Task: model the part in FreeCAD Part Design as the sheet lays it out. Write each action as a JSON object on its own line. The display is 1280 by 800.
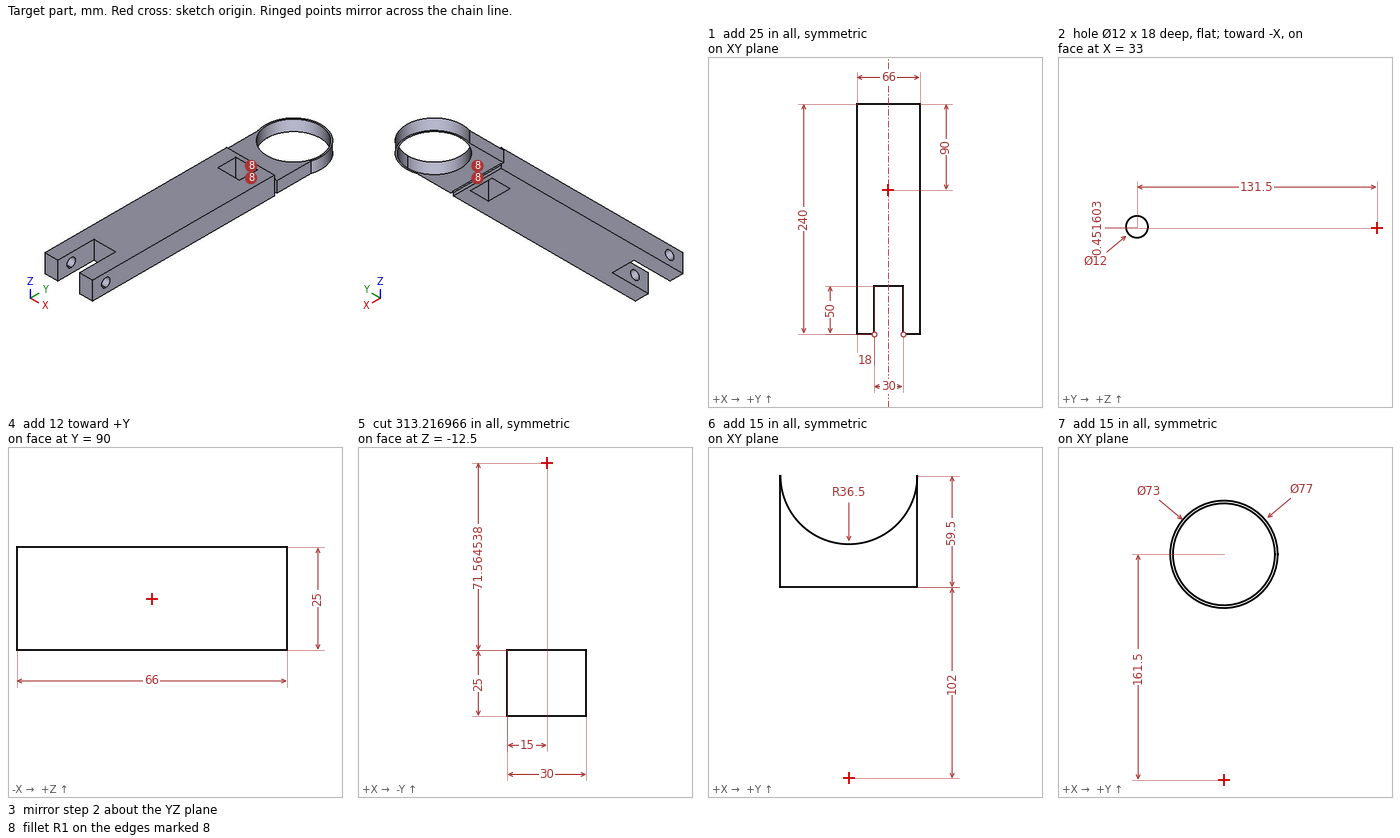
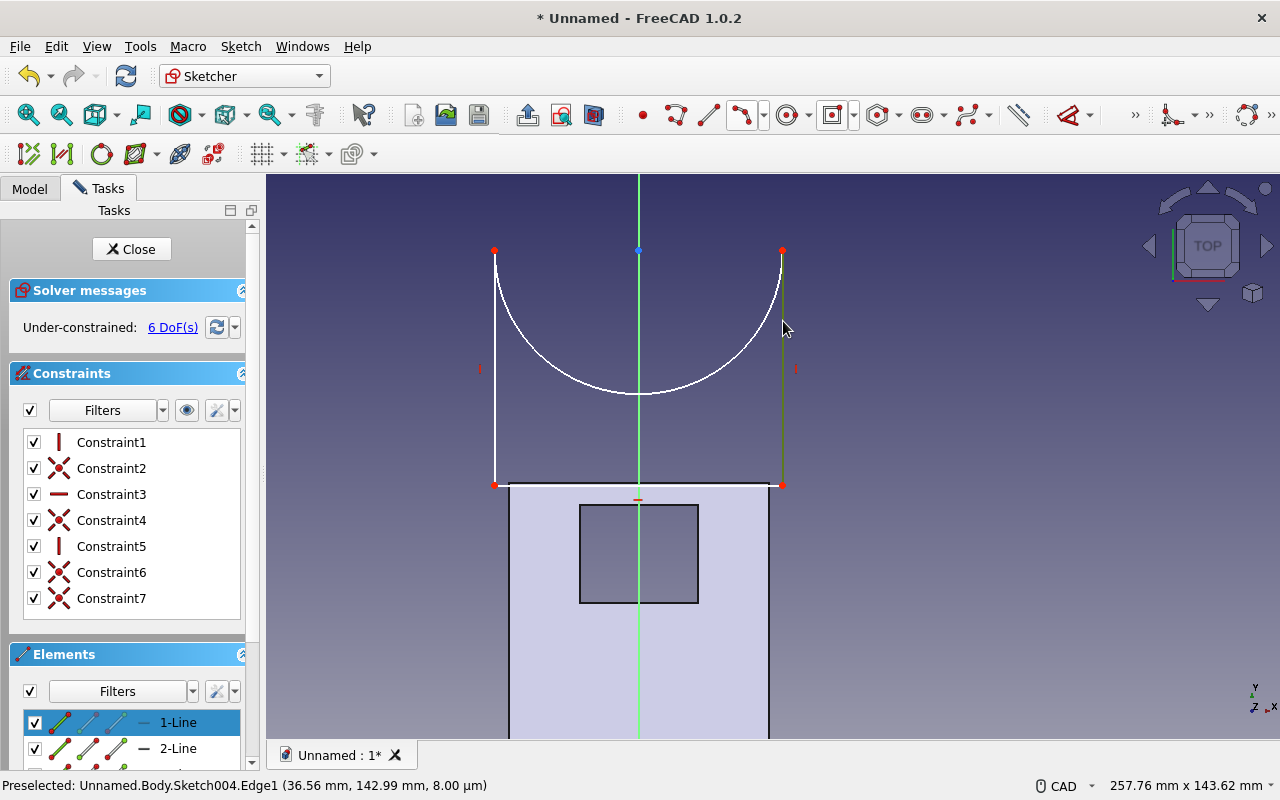
{"action": "left_click", "coordinate": [554, 367]}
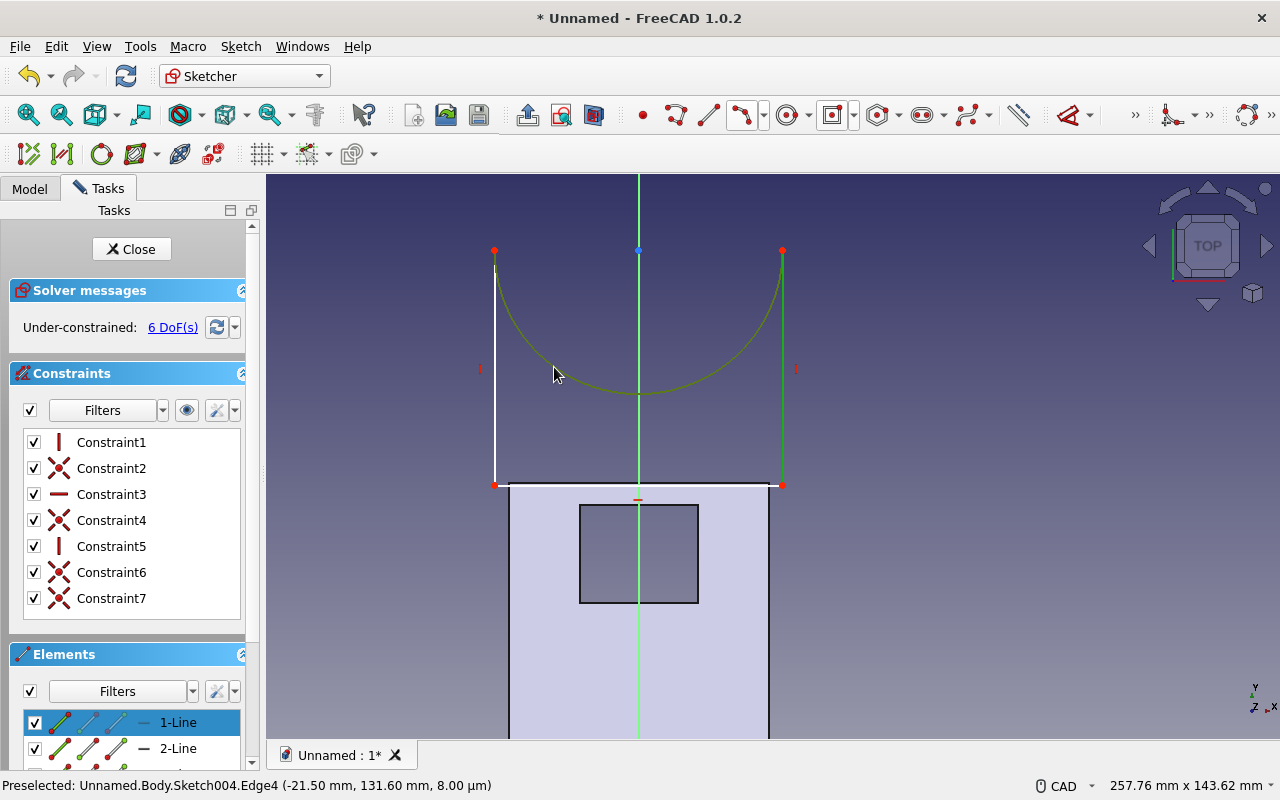
{"action": "key", "text": "t"}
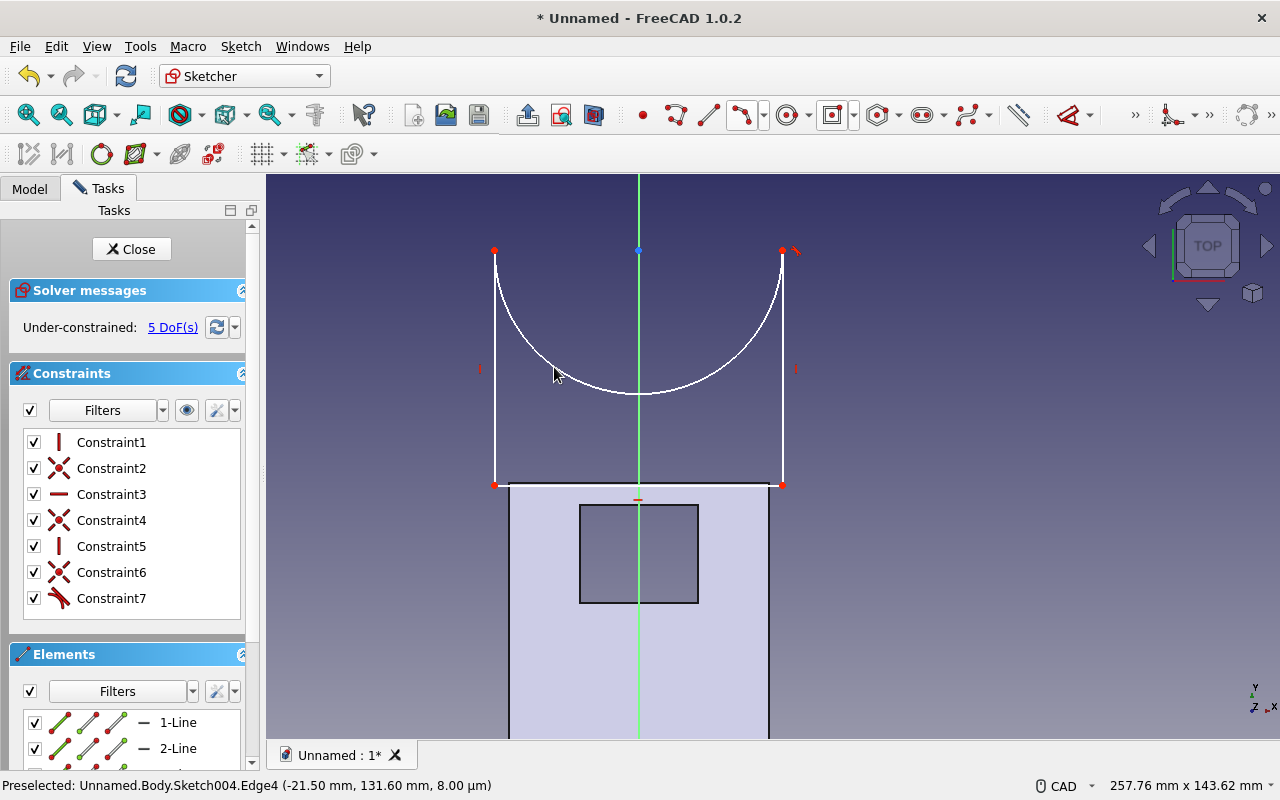
{"action": "left_click", "coordinate": [495, 415]}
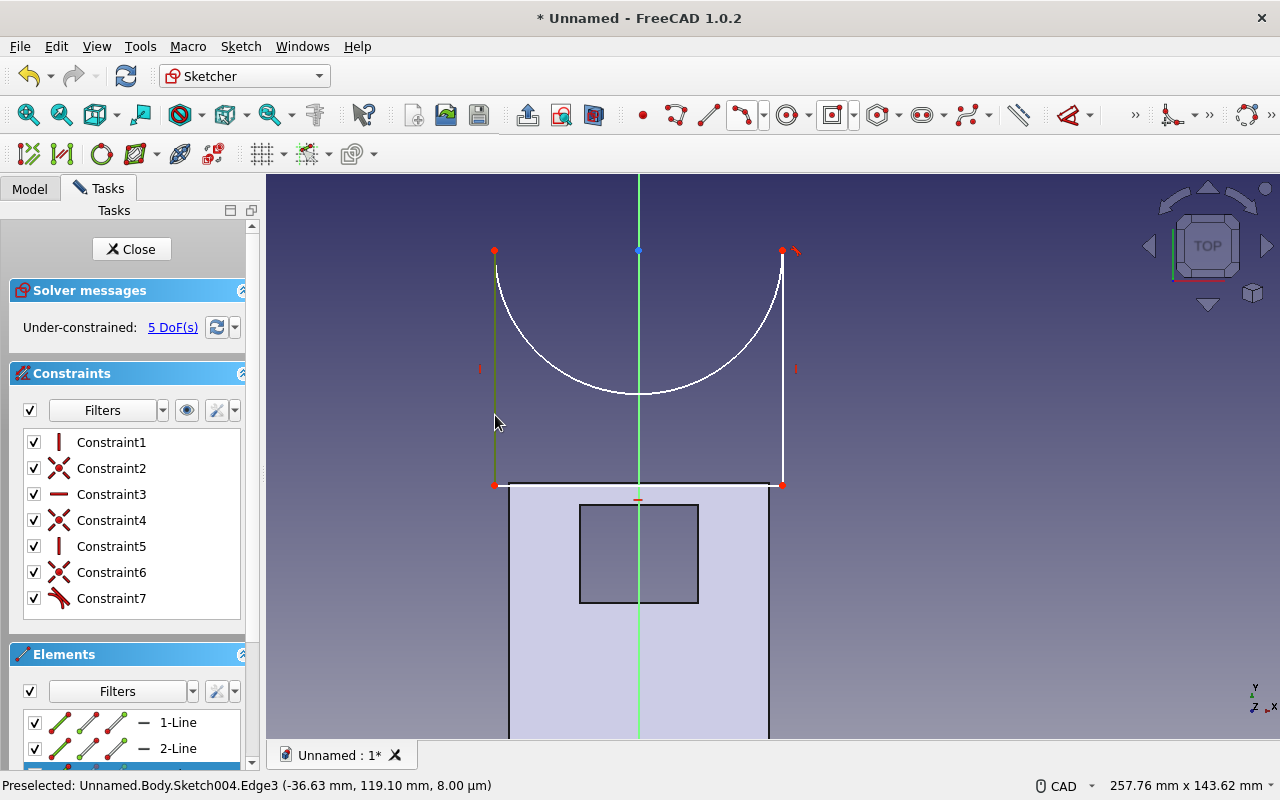
{"action": "left_click", "coordinate": [554, 367]}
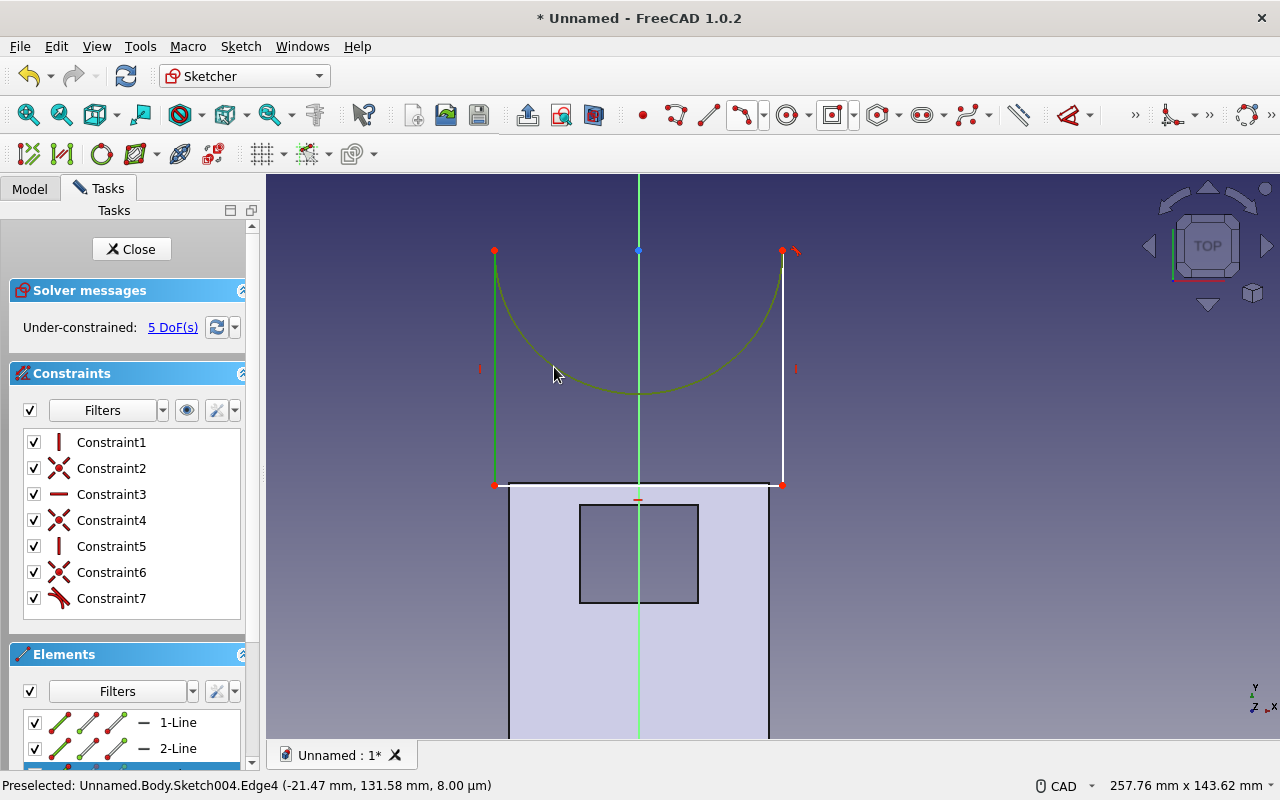
{"action": "key", "text": "t"}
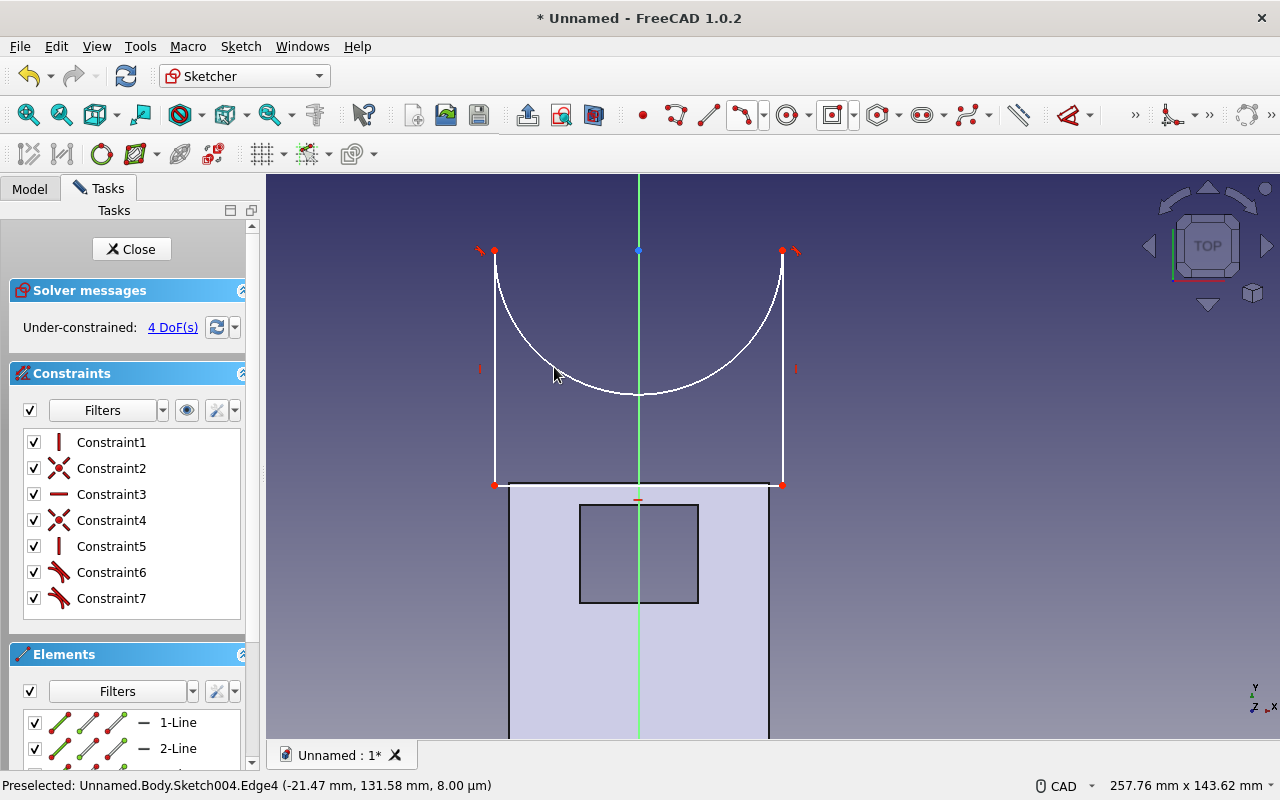
{"action": "left_click", "coordinate": [639, 251]}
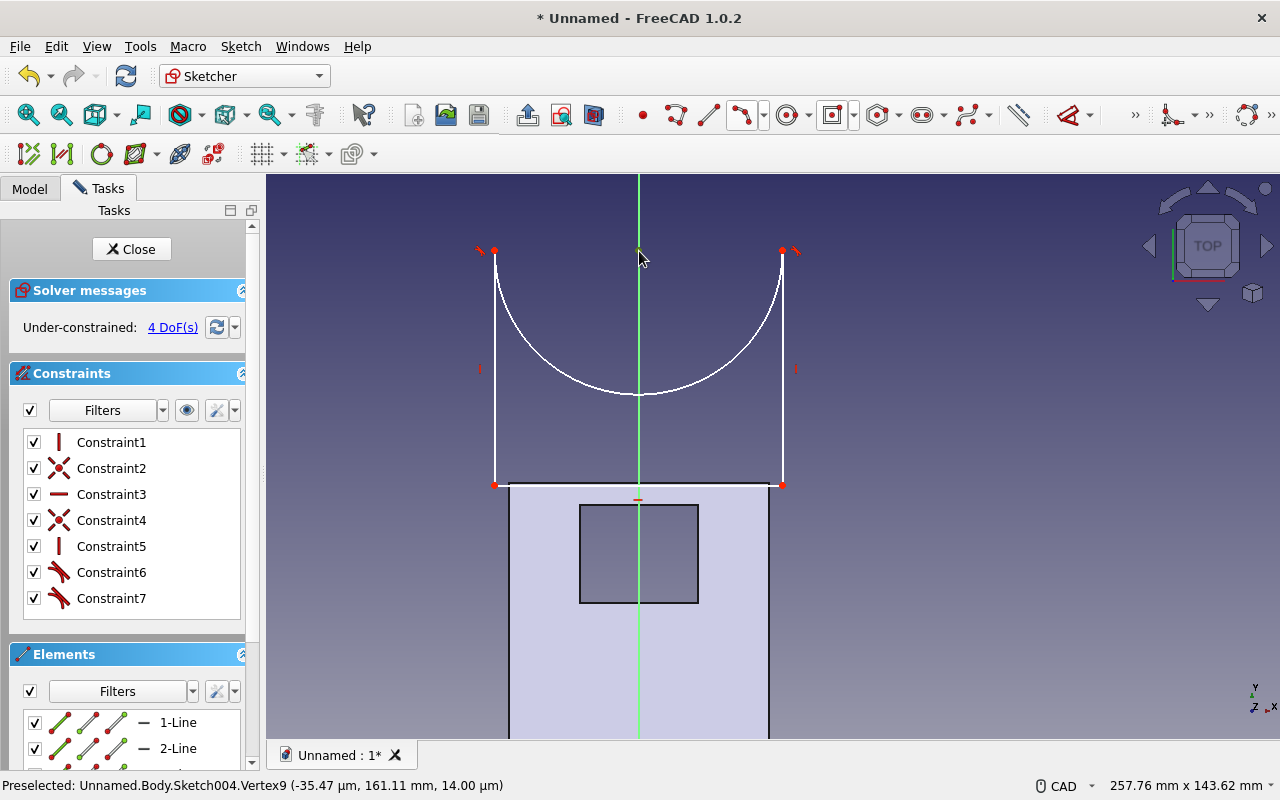
{"action": "left_click", "coordinate": [639, 675]}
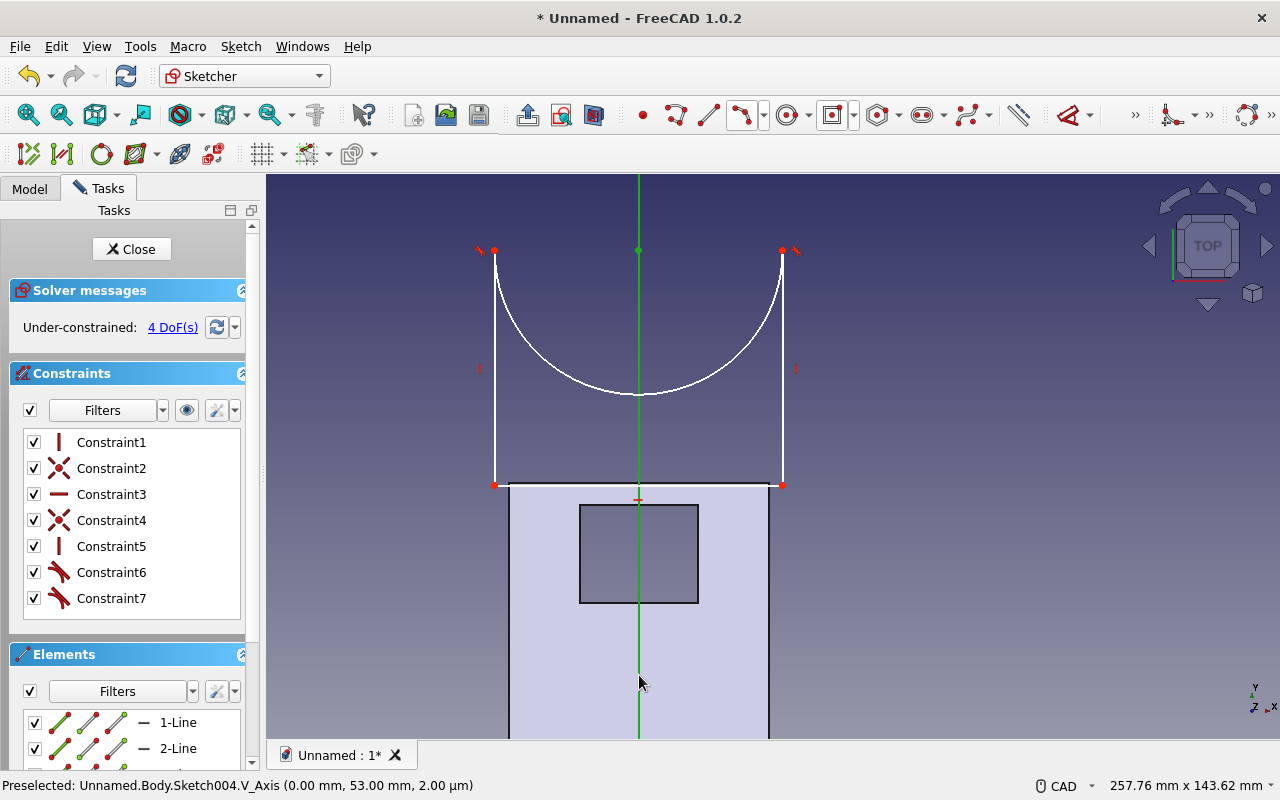
{"action": "key", "text": "c"}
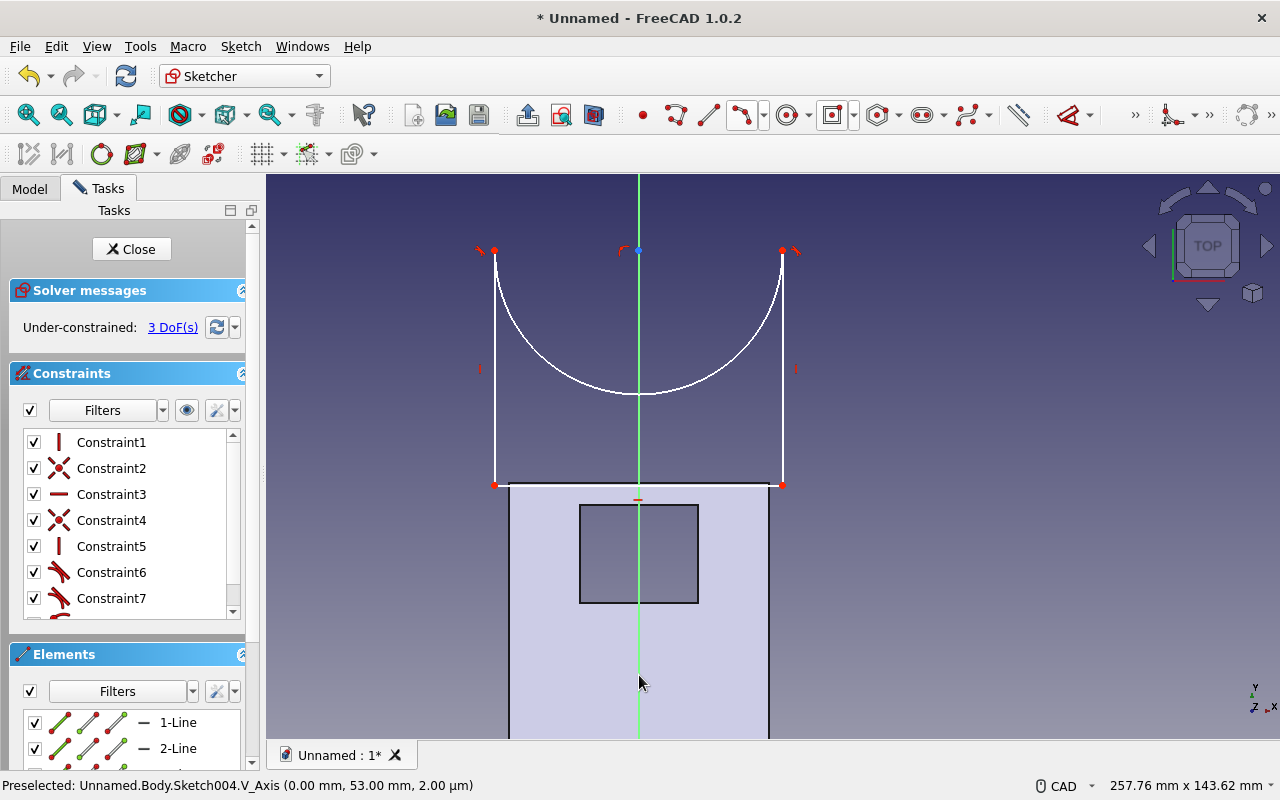
{"action": "left_click", "coordinate": [1068, 116]}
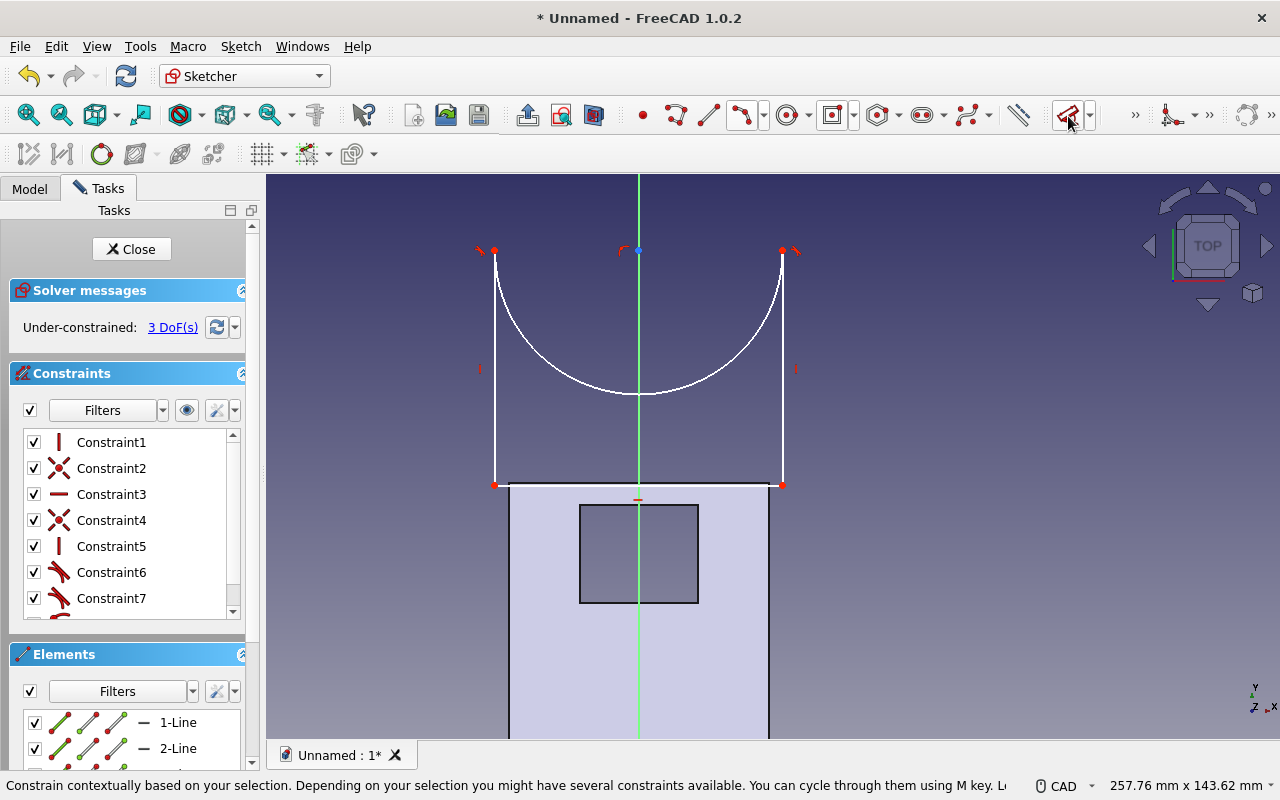
{"action": "left_click", "coordinate": [554, 367]}
{"action": "left_click", "coordinate": [535, 393]}